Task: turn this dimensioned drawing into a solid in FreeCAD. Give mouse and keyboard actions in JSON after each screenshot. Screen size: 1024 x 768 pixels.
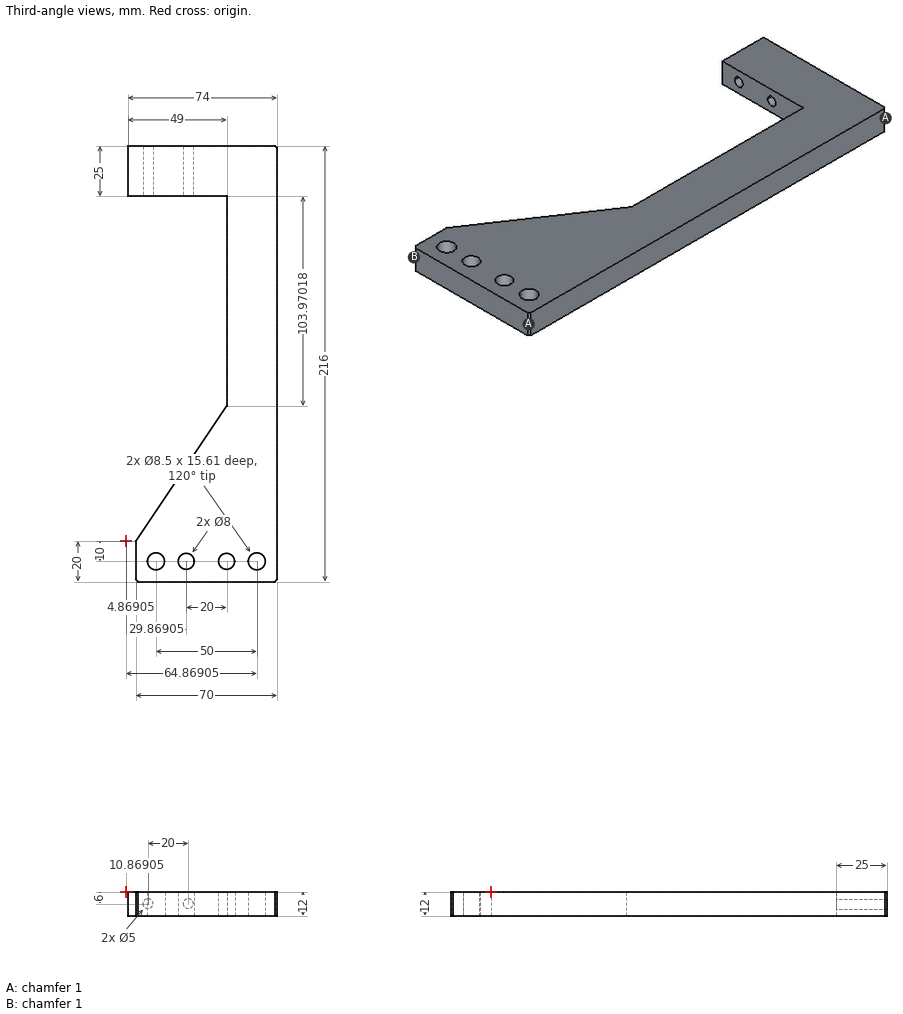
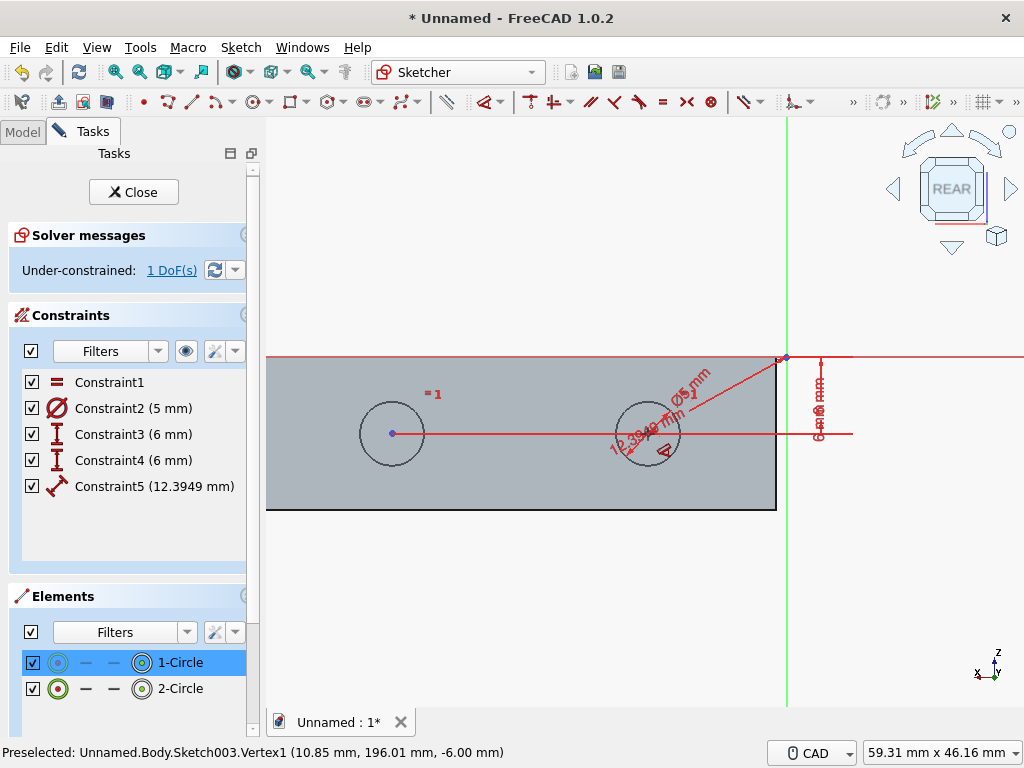
{"action": "left_click", "coordinate": [392, 434]}
{"action": "left_click", "coordinate": [520, 468]}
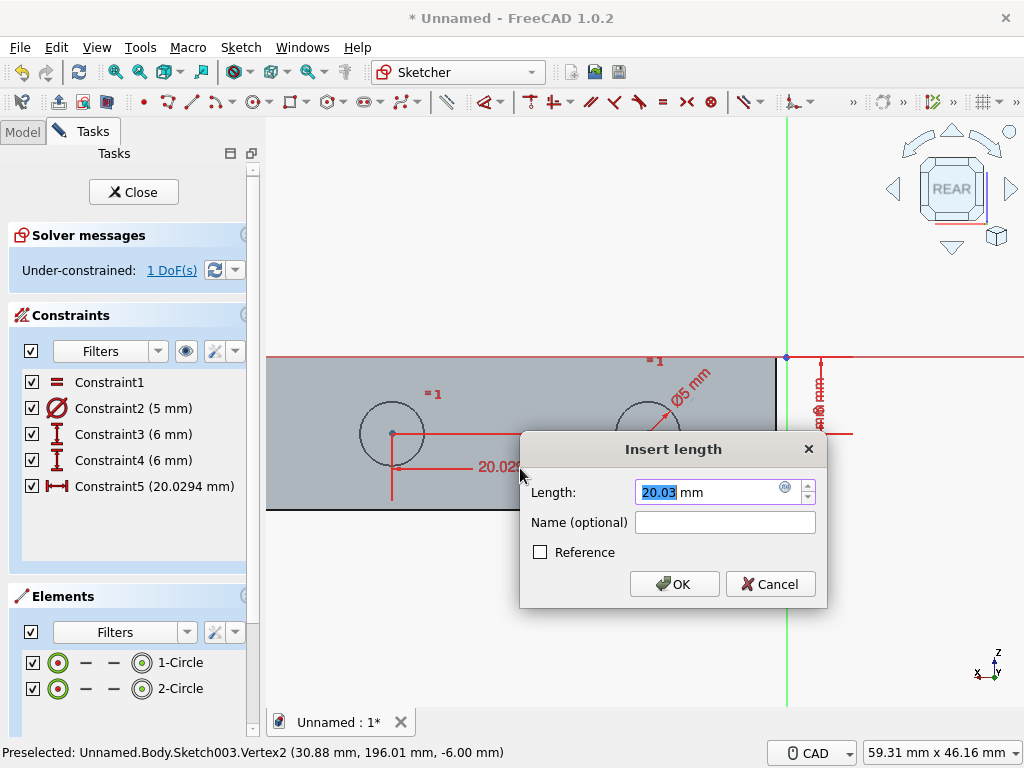
{"action": "type", "text": "20"}
{"action": "key", "text": "Return"}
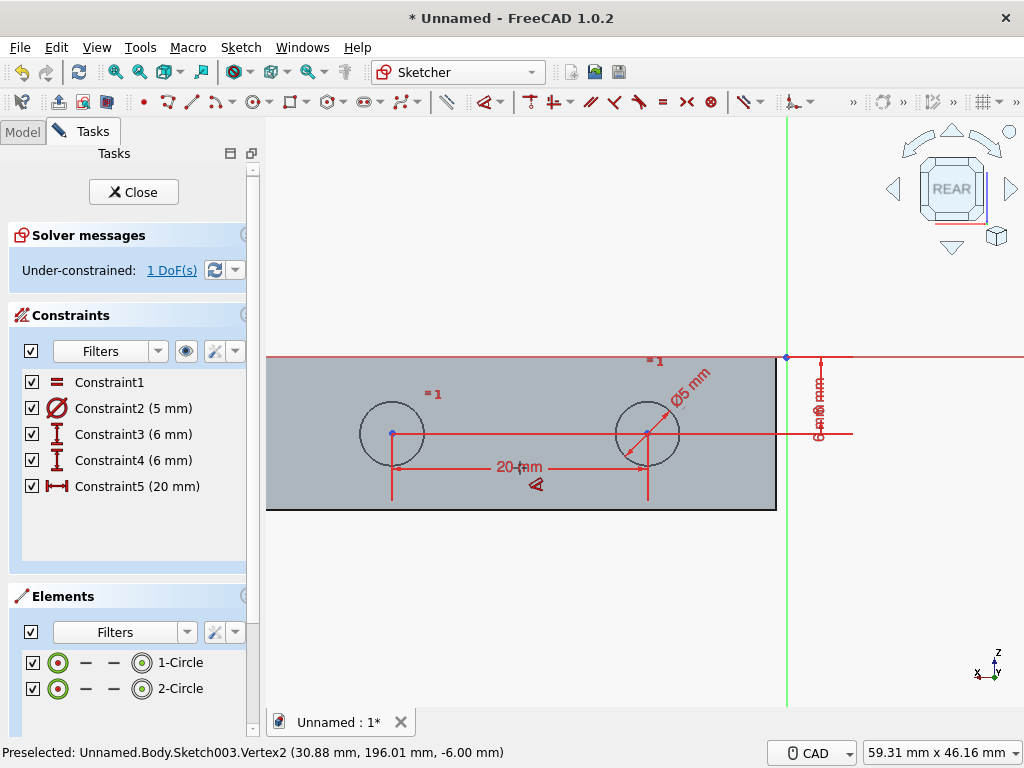
{"action": "left_click", "coordinate": [648, 434]}
{"action": "left_click", "coordinate": [717, 323]}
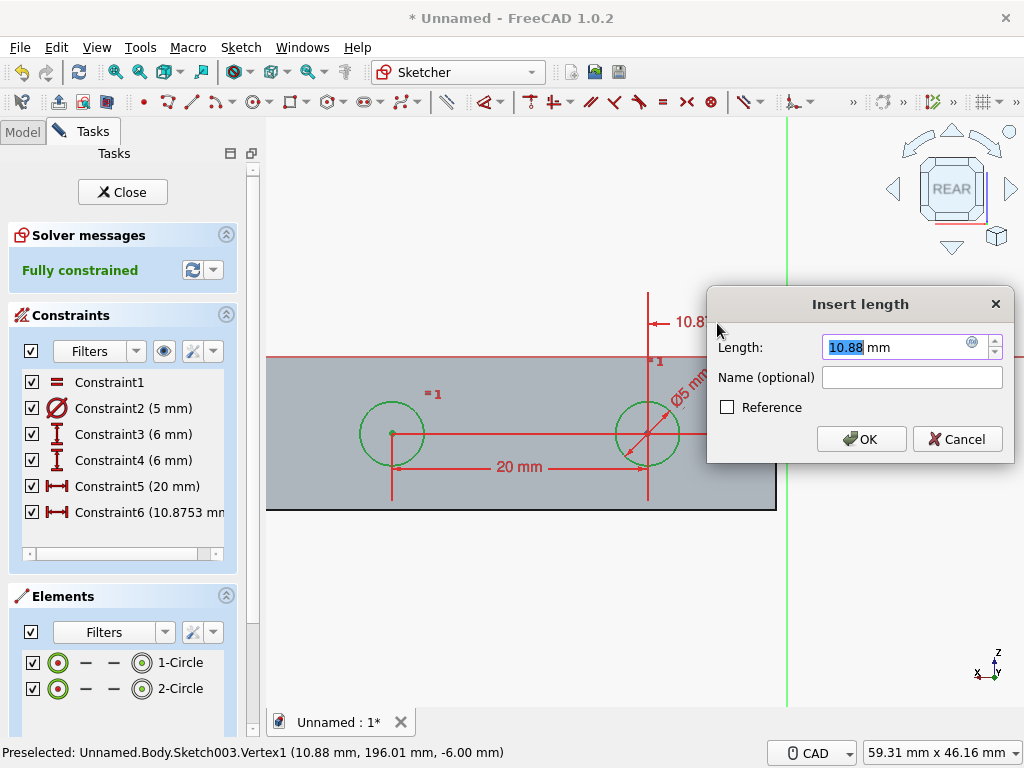
{"action": "type", "text": "10.86905"}
{"action": "key", "text": "Return"}
{"action": "key", "text": "Escape"}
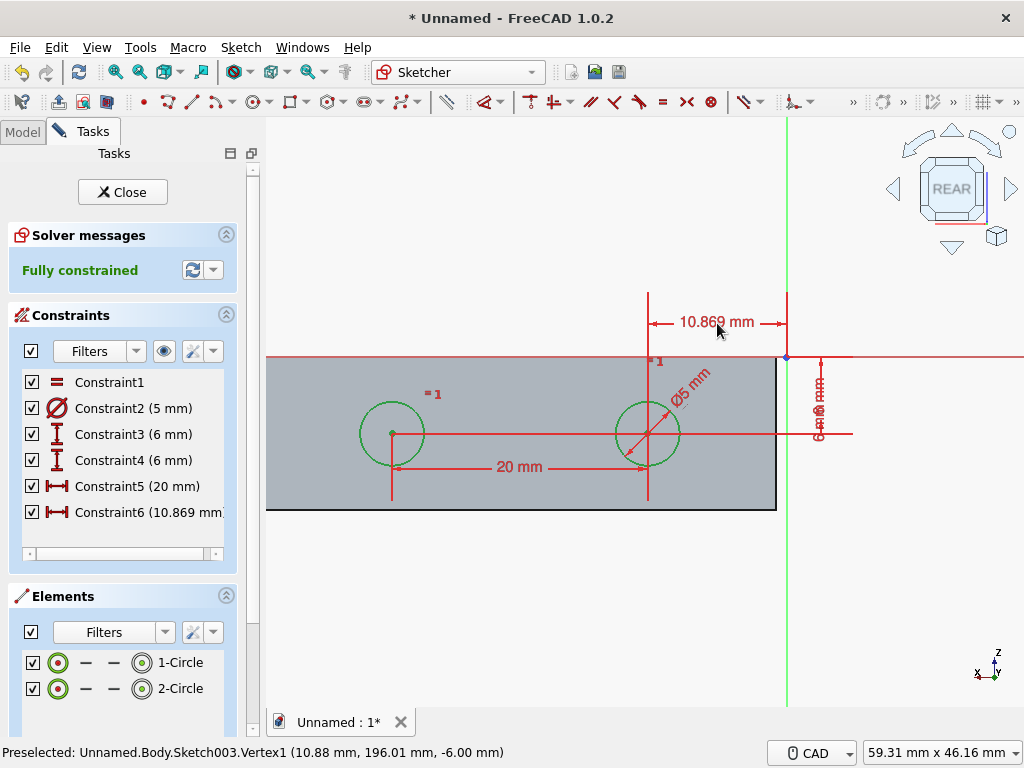
{"action": "left_click", "coordinate": [123, 192]}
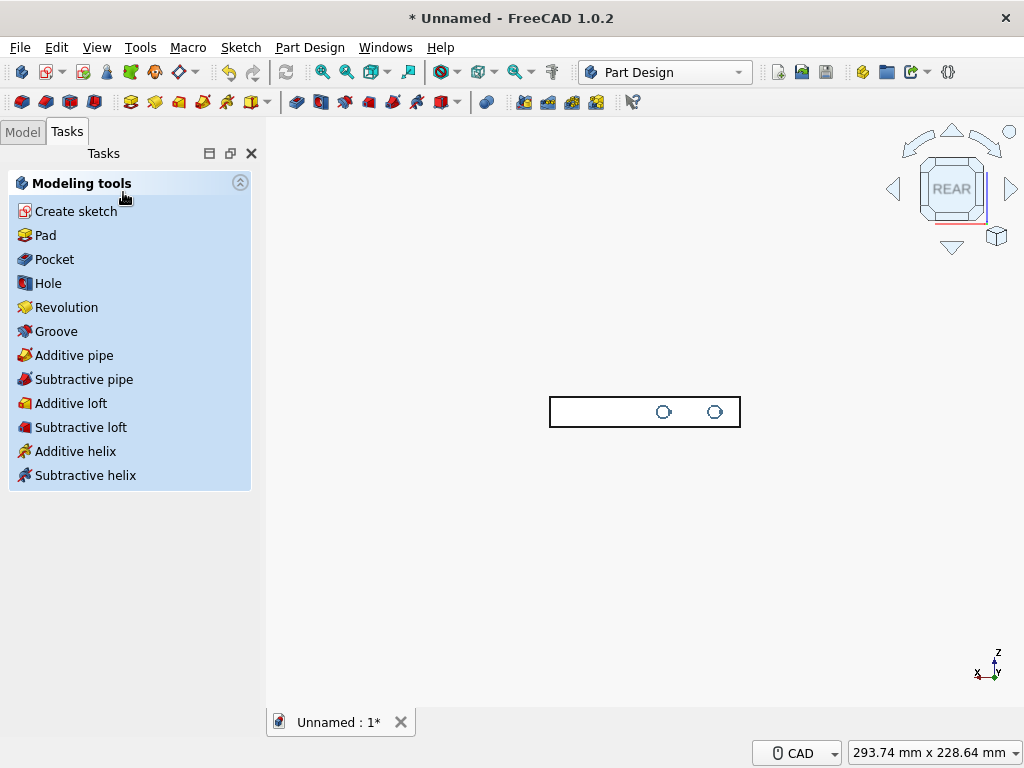
{"action": "left_click", "coordinate": [298, 102]}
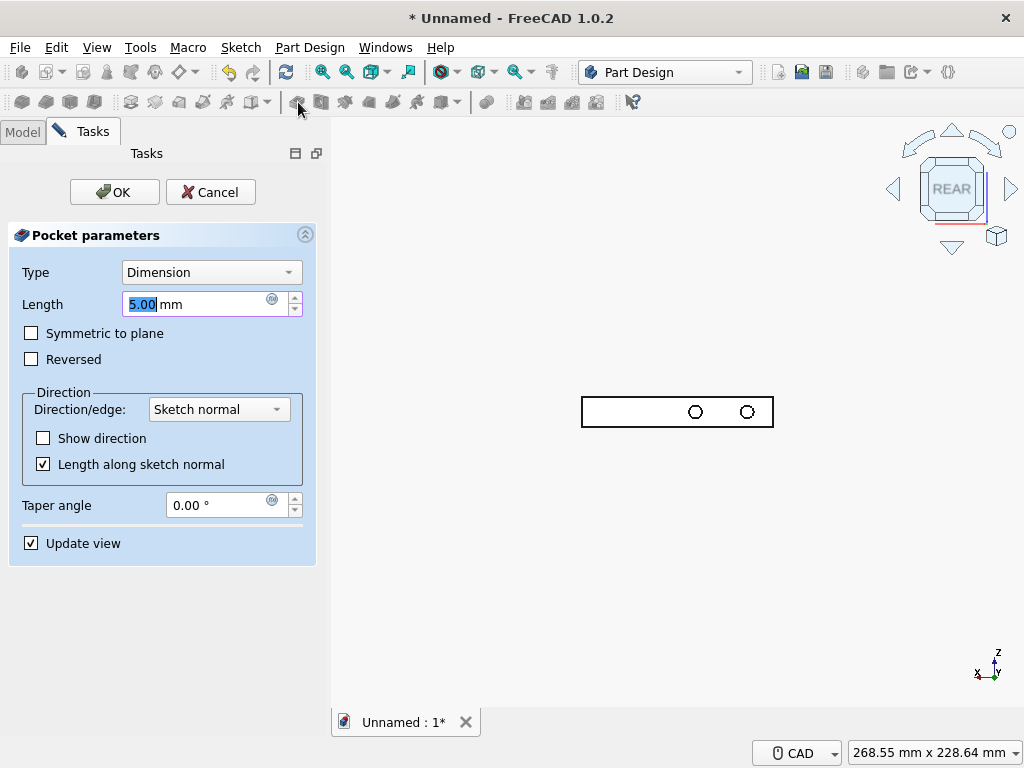
{"action": "type", "text": "25"}
{"action": "key", "text": "Tab"}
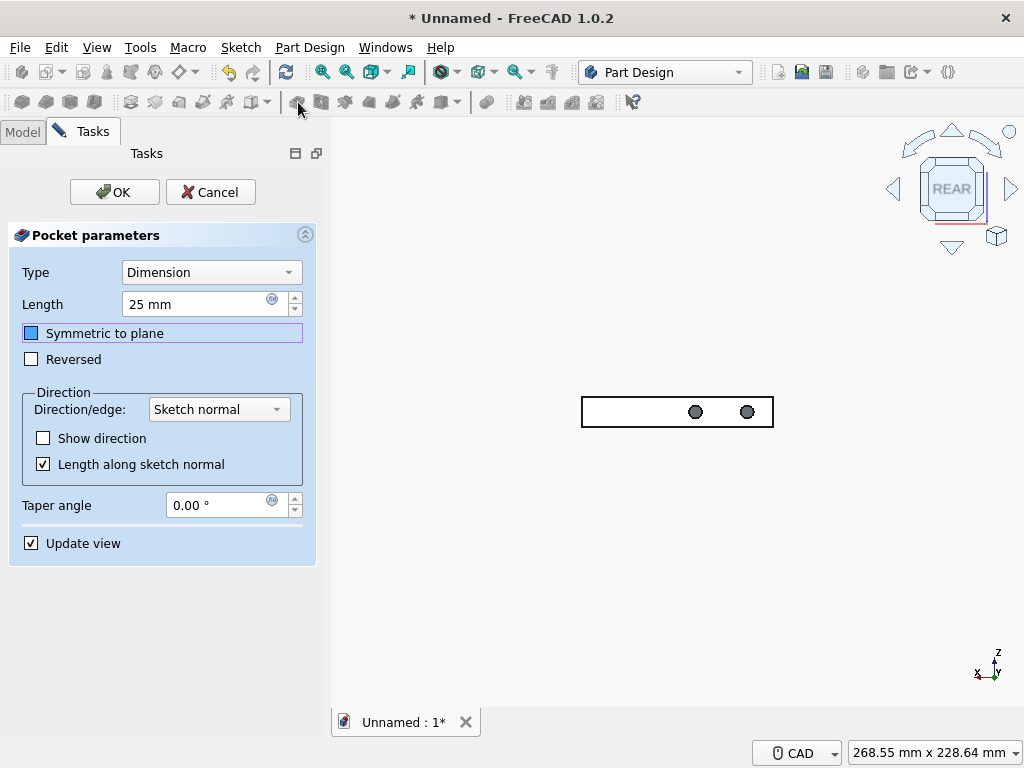
{"action": "left_click", "coordinate": [115, 192]}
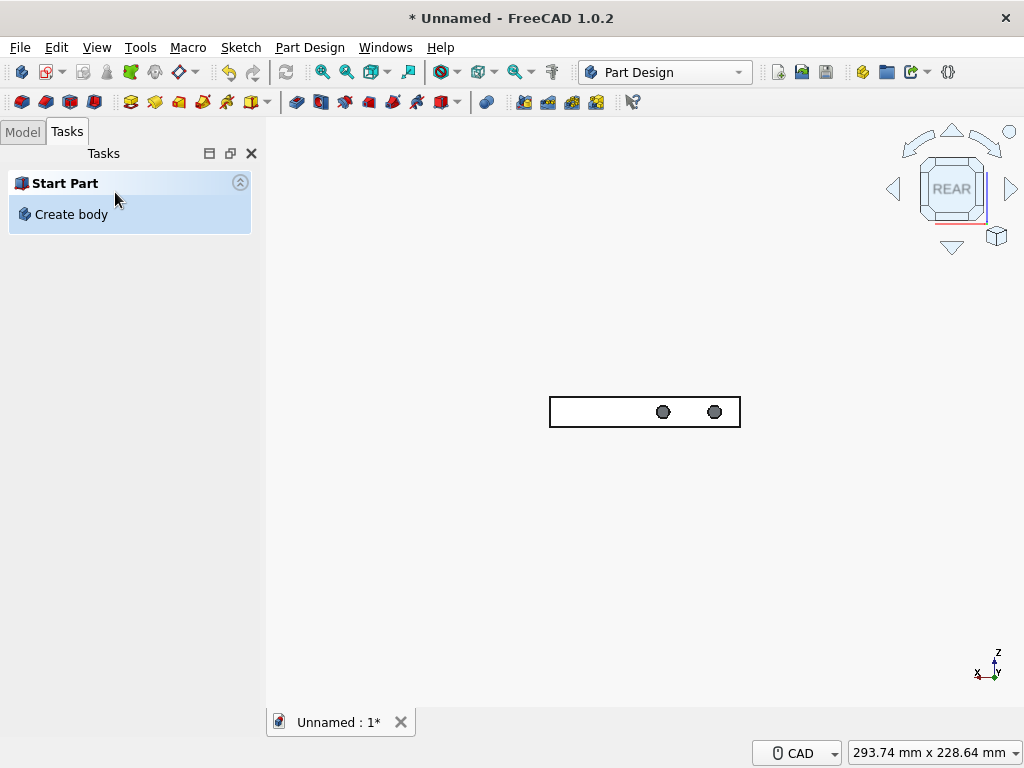
{"action": "key", "text": "v f"}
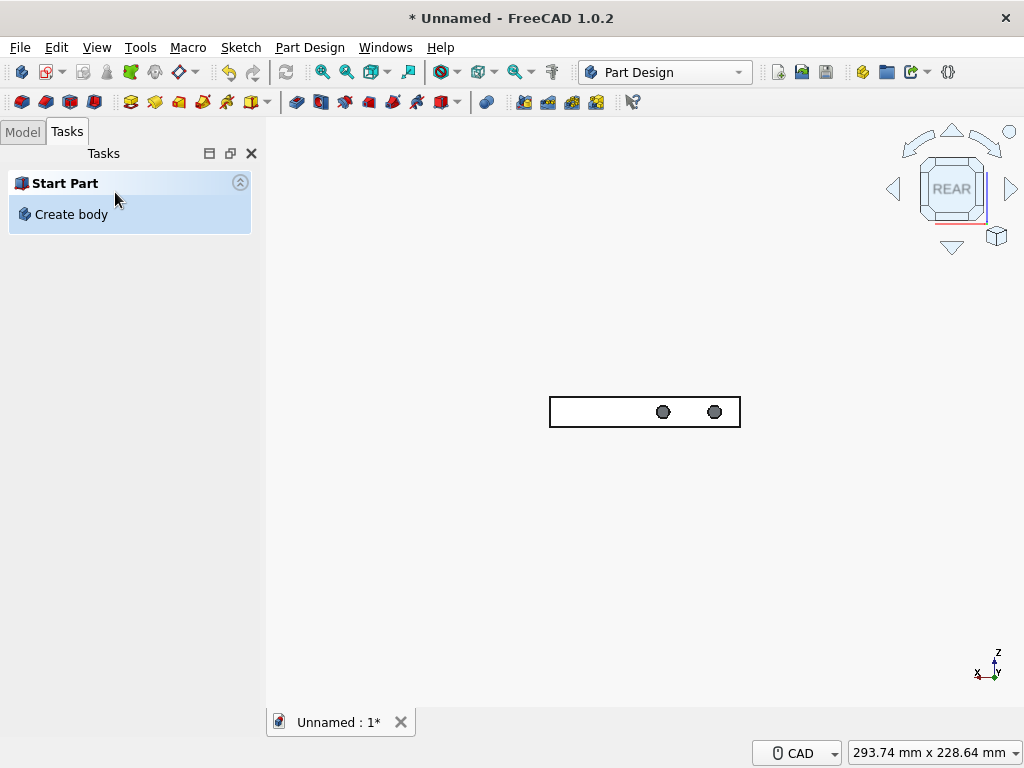
{"action": "key", "text": "0"}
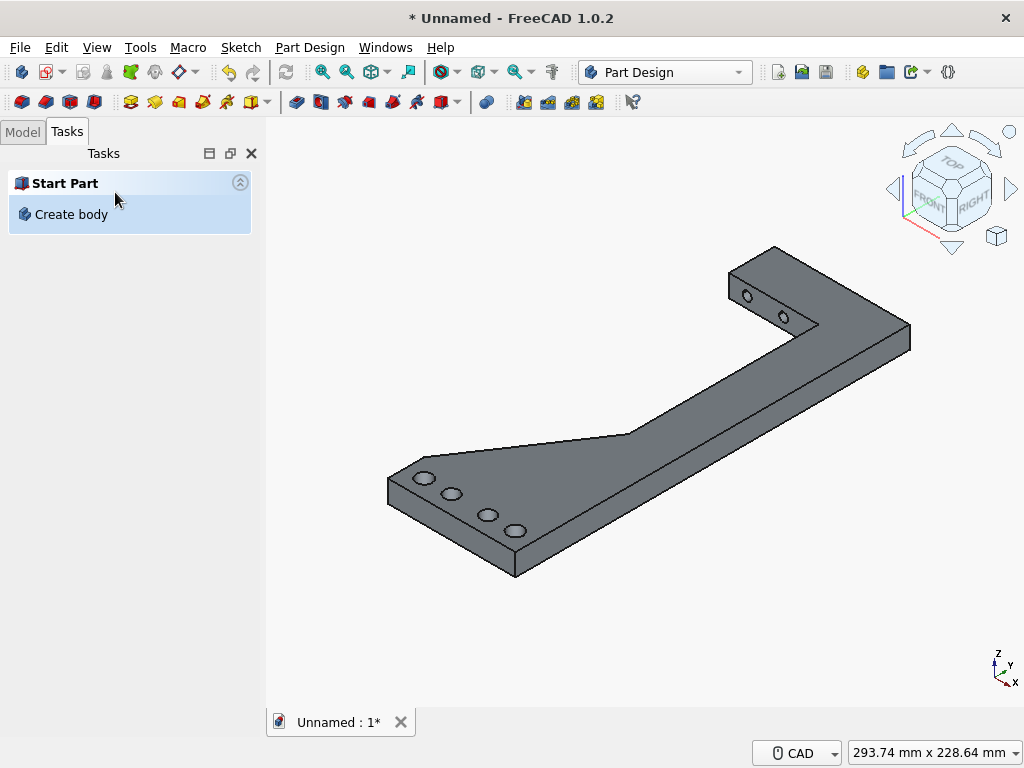
{"action": "left_click", "coordinate": [515, 564]}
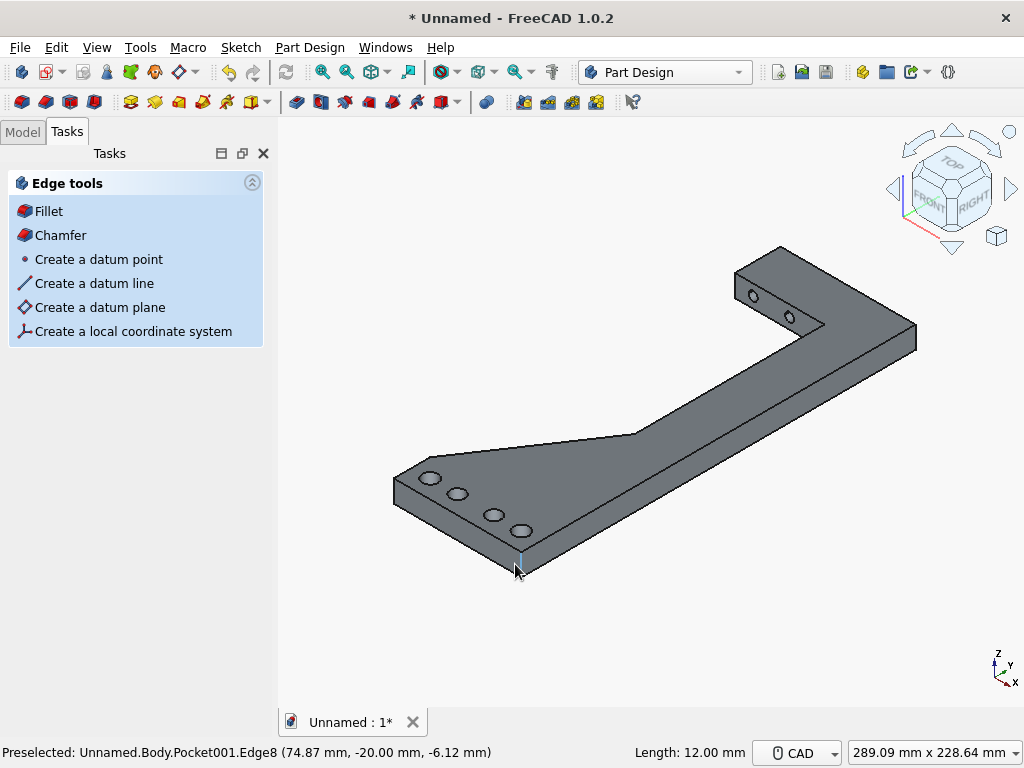
{"action": "key", "text": "2"}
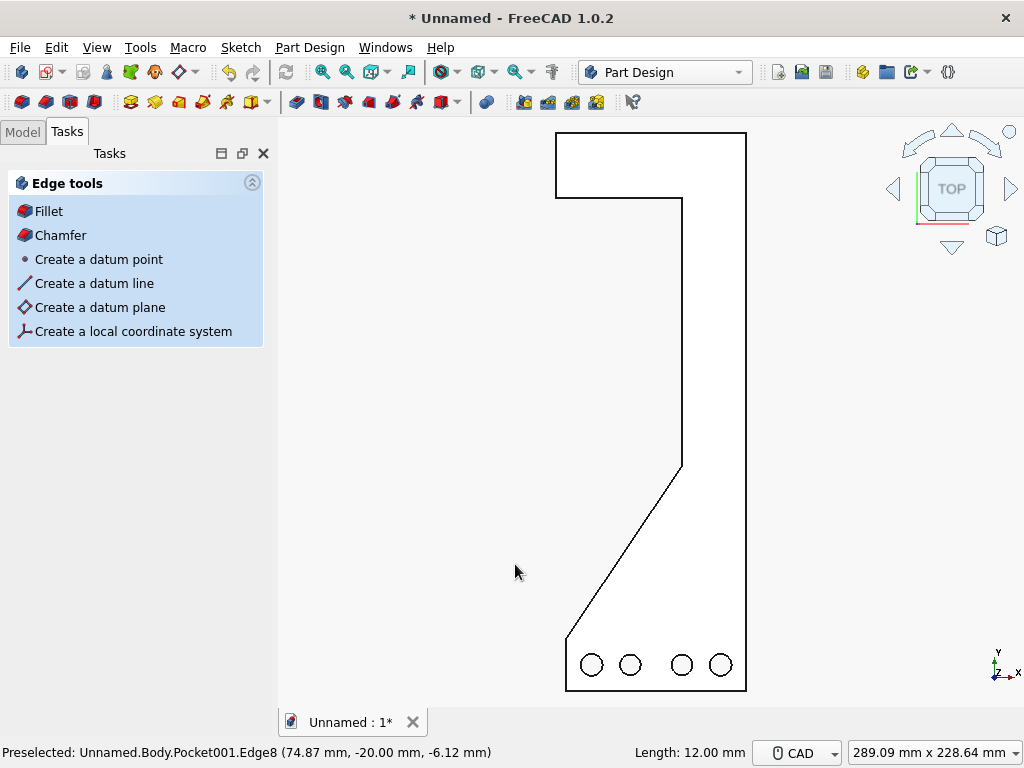
{"action": "key", "text": "1"}